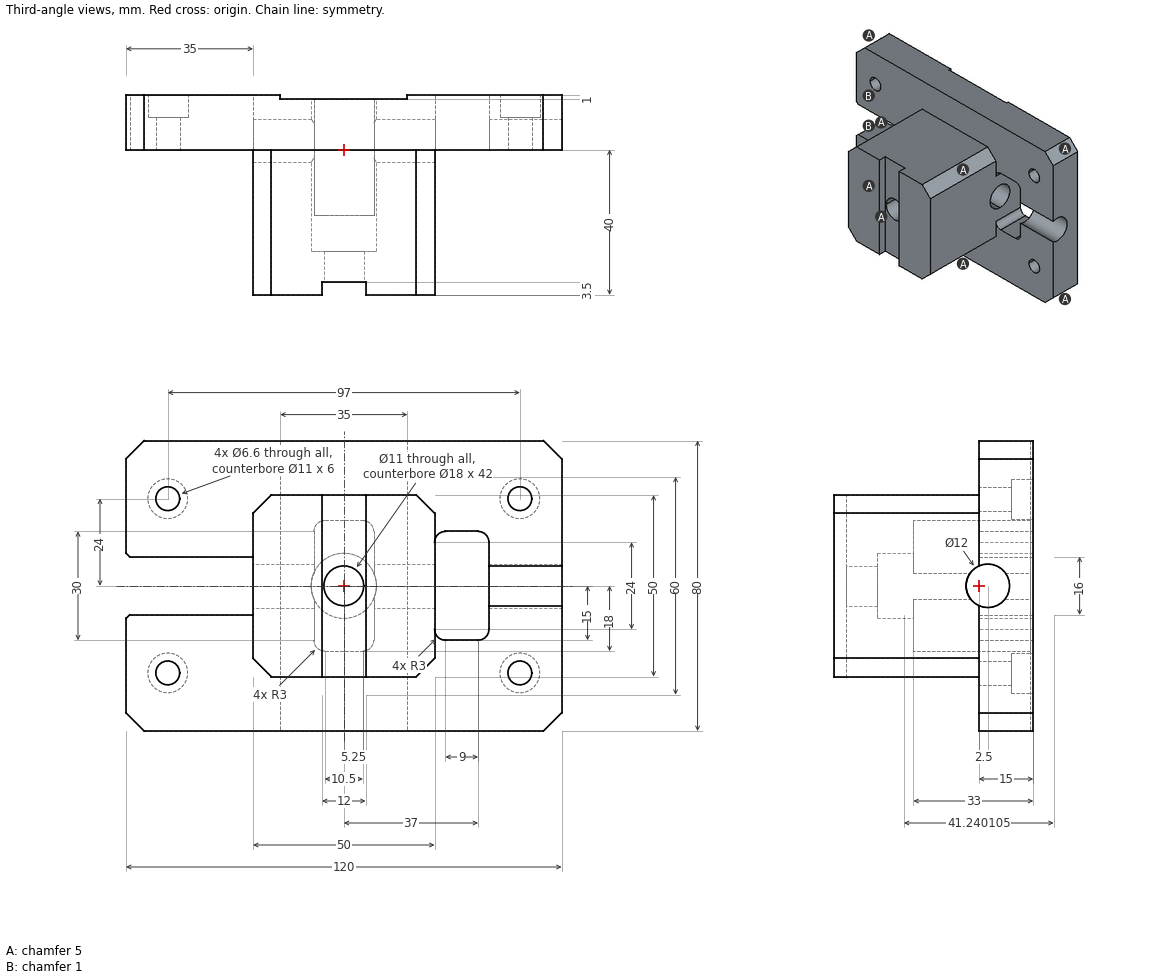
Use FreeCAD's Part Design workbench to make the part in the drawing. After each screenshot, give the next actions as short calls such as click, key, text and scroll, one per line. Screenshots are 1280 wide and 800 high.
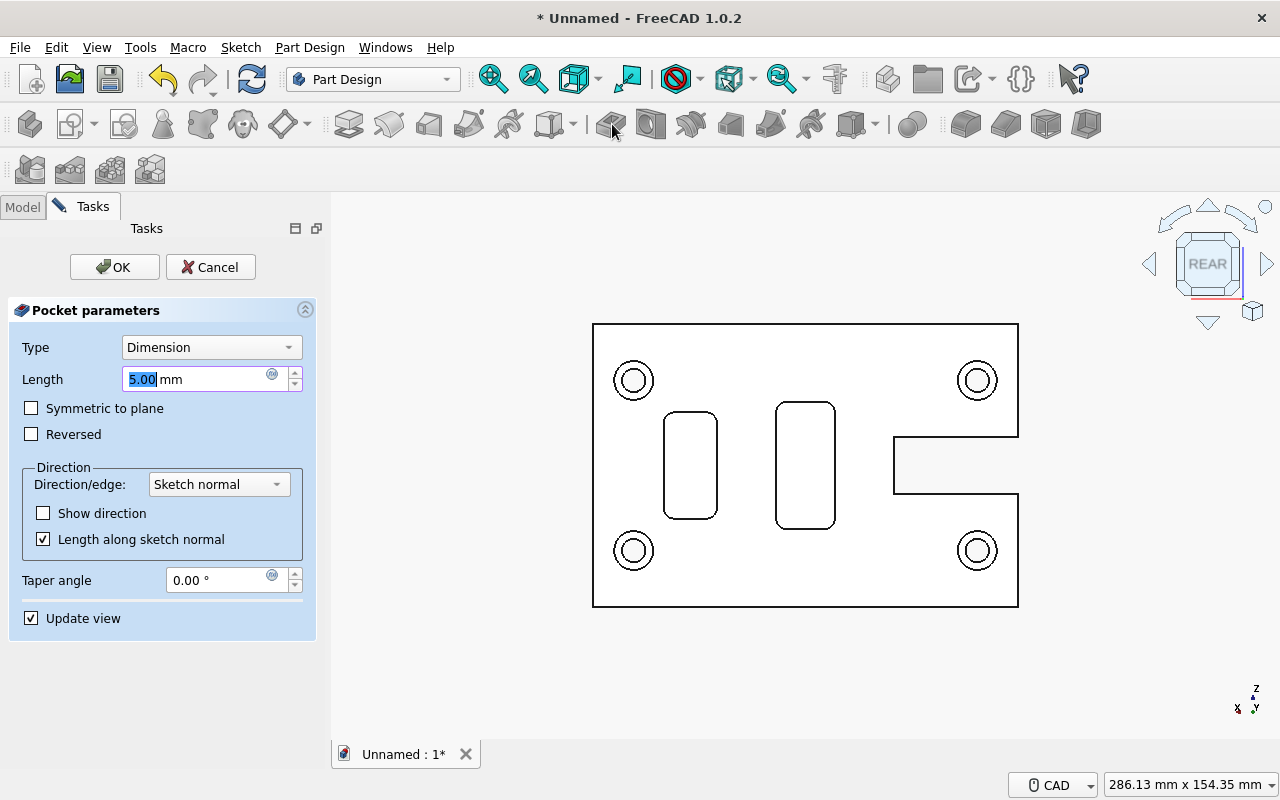
click(212, 348)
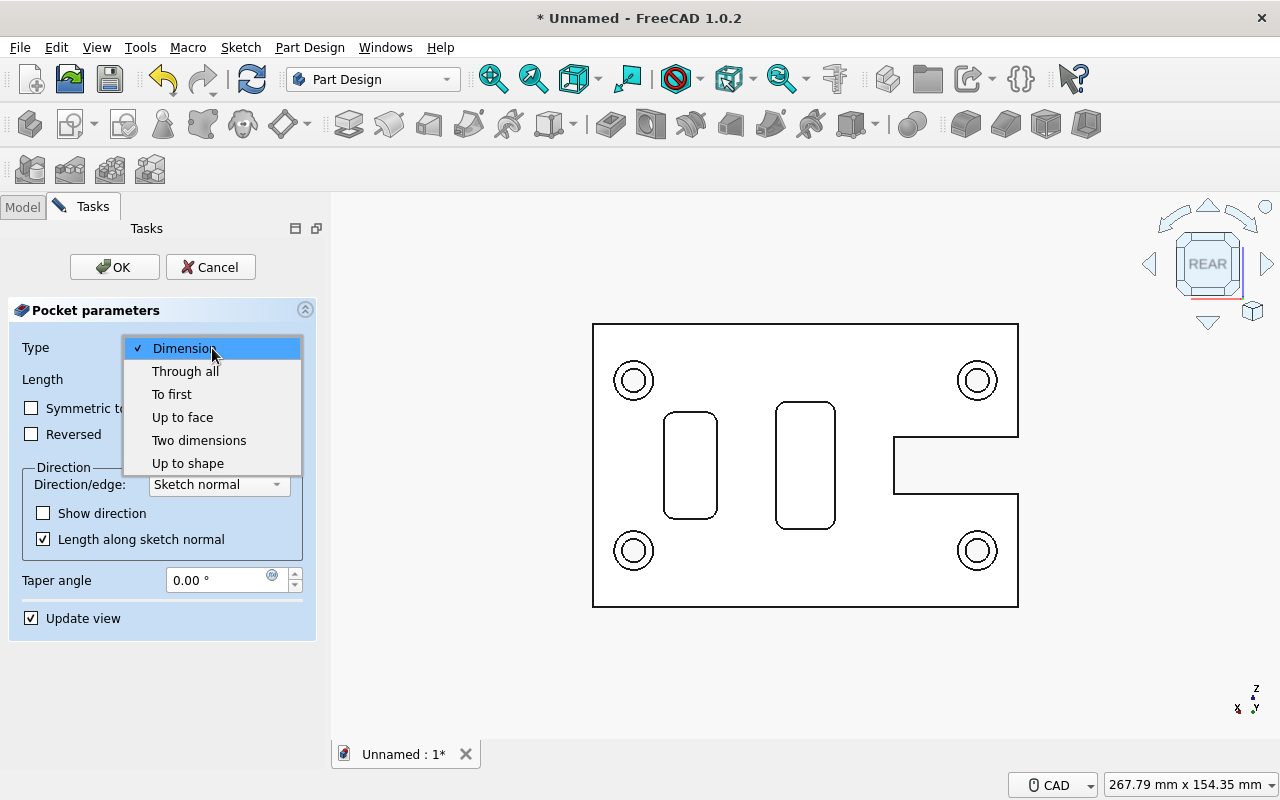
click(212, 372)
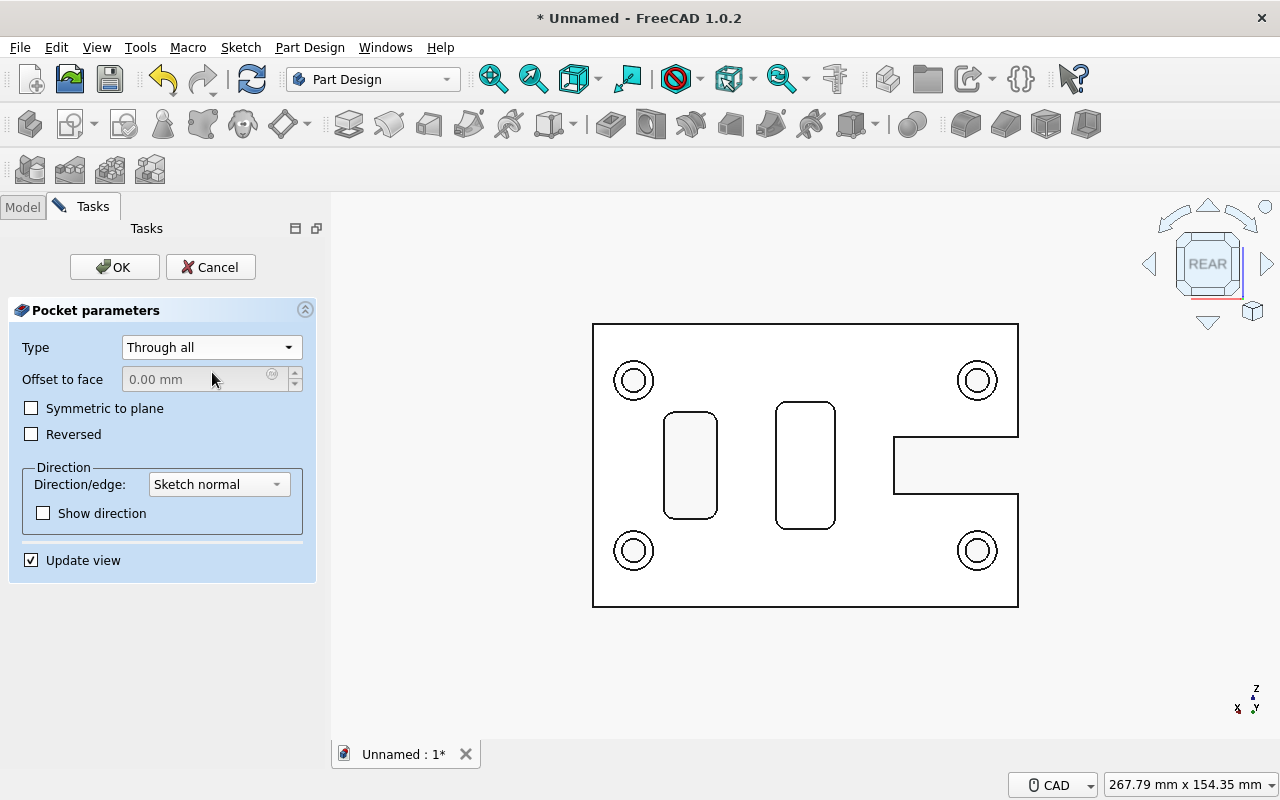
click(115, 267)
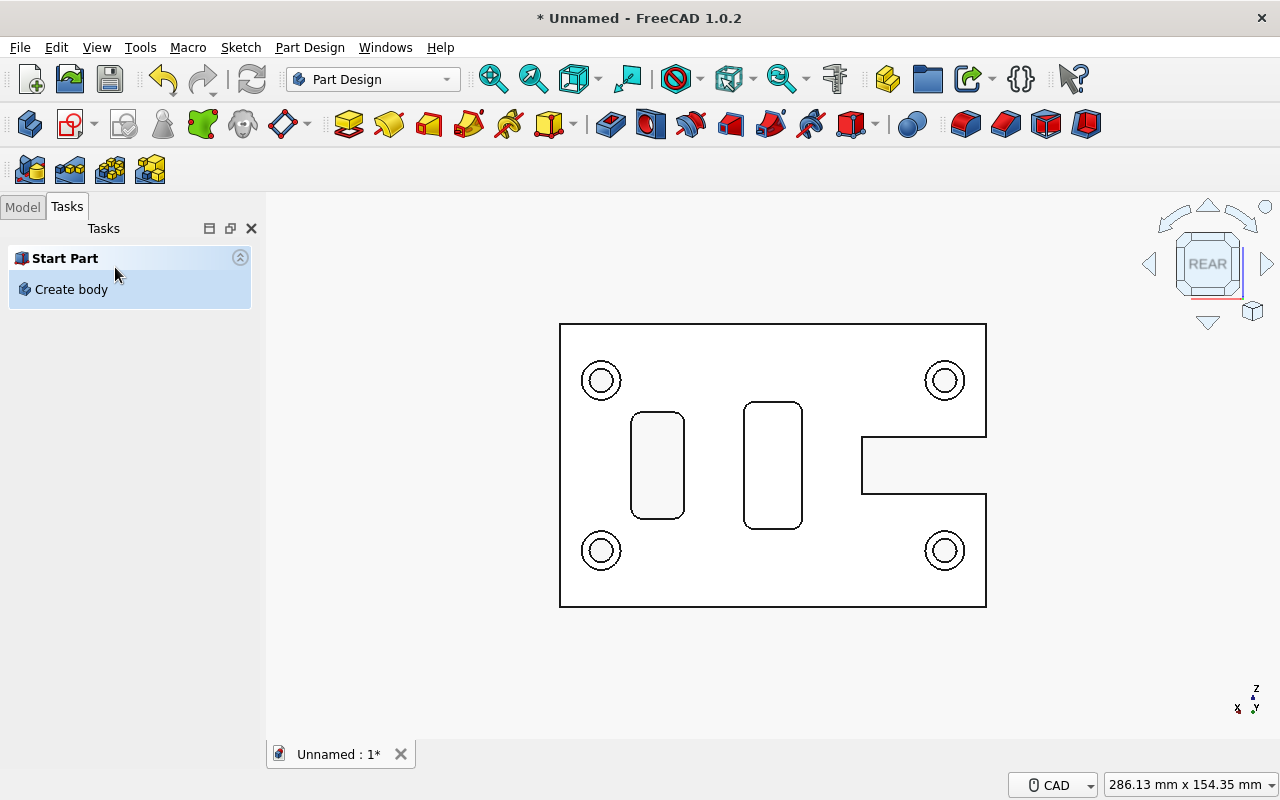
key(0)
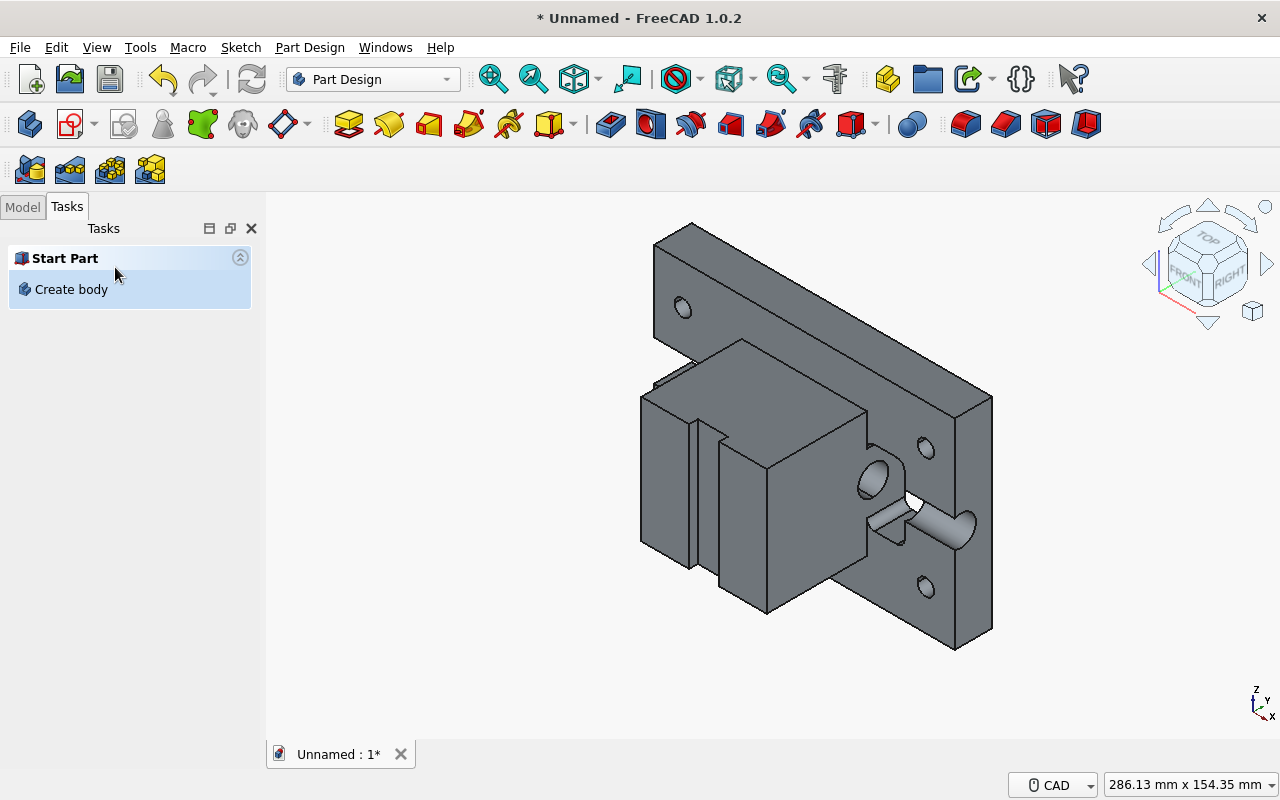
click(817, 439)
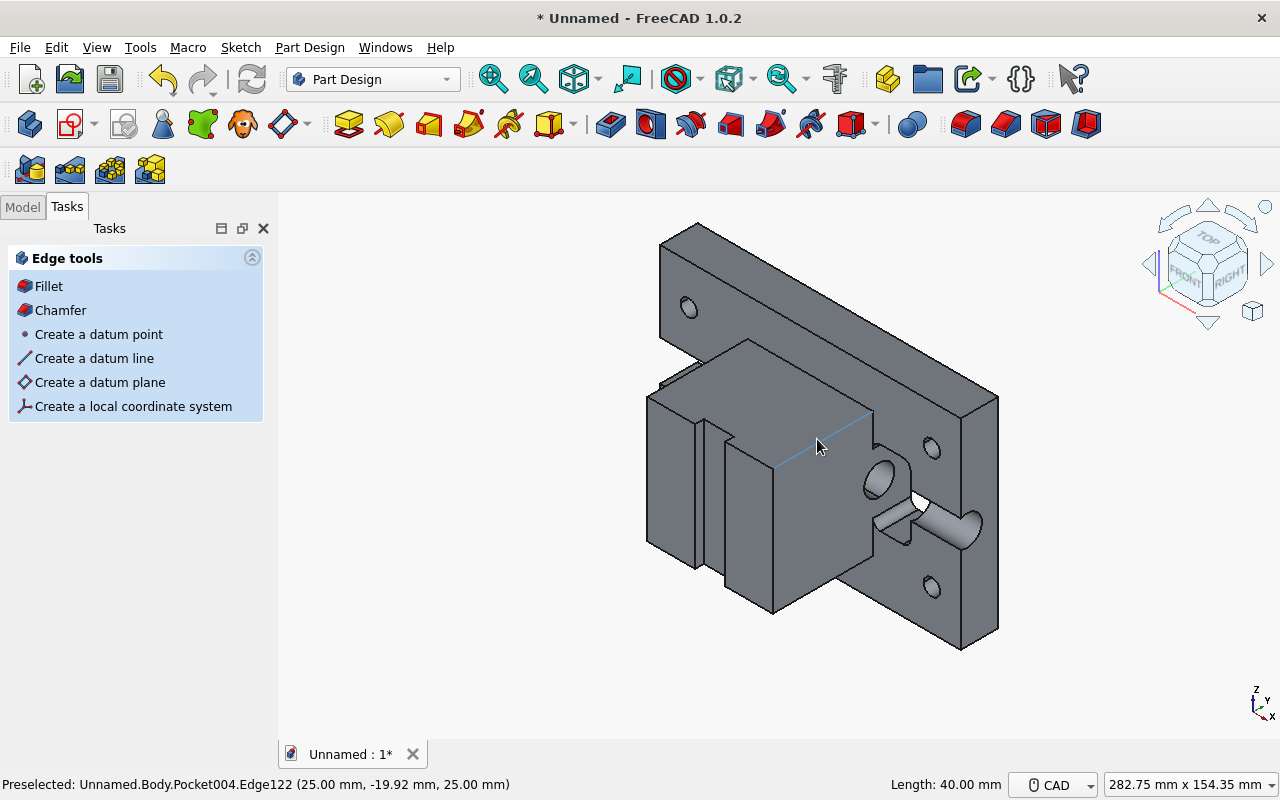
click(979, 407, ctrl)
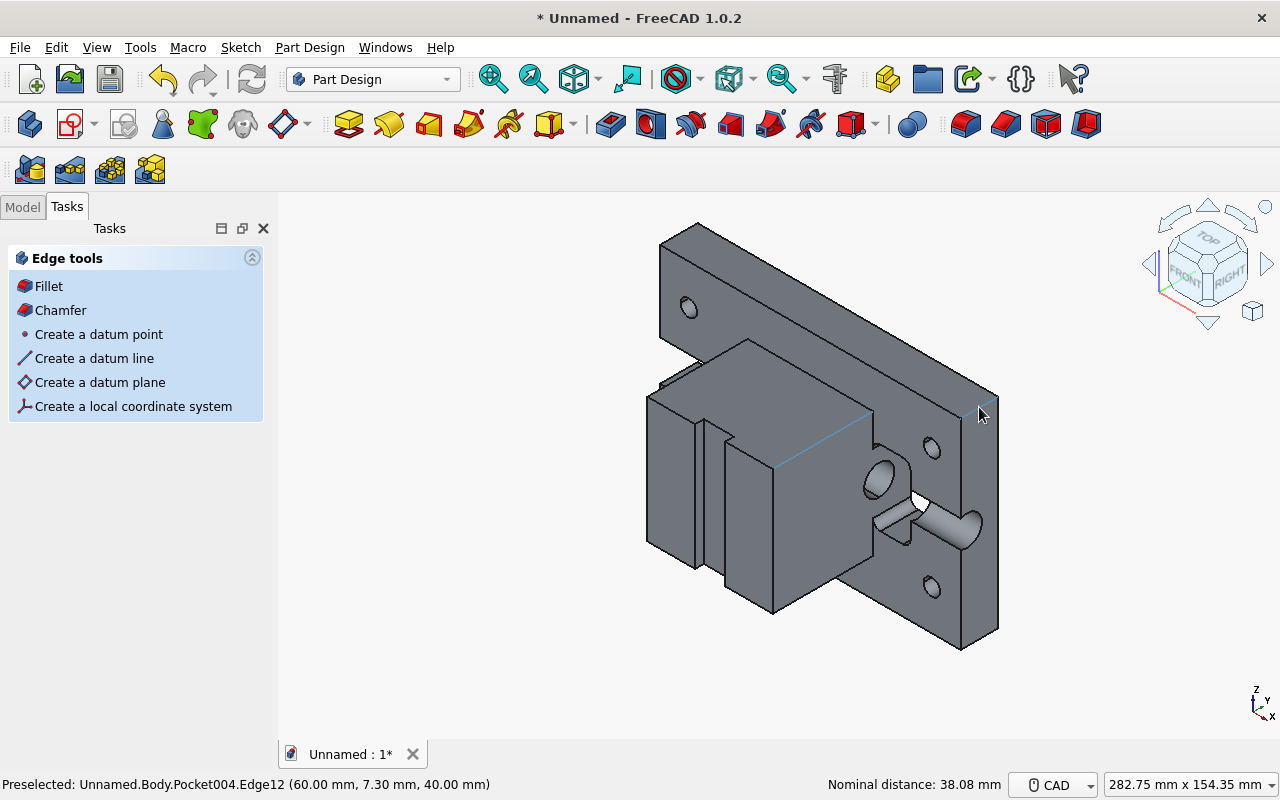
key(2)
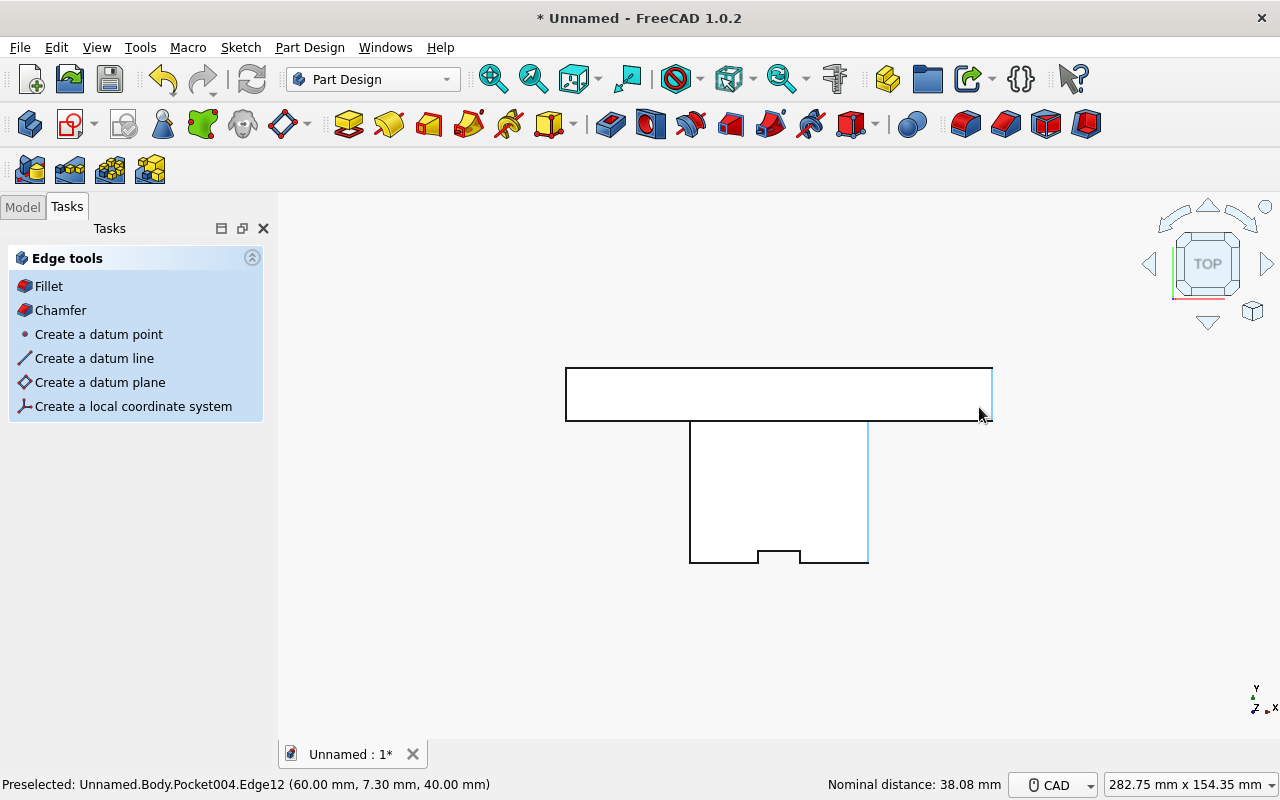
click(494, 80)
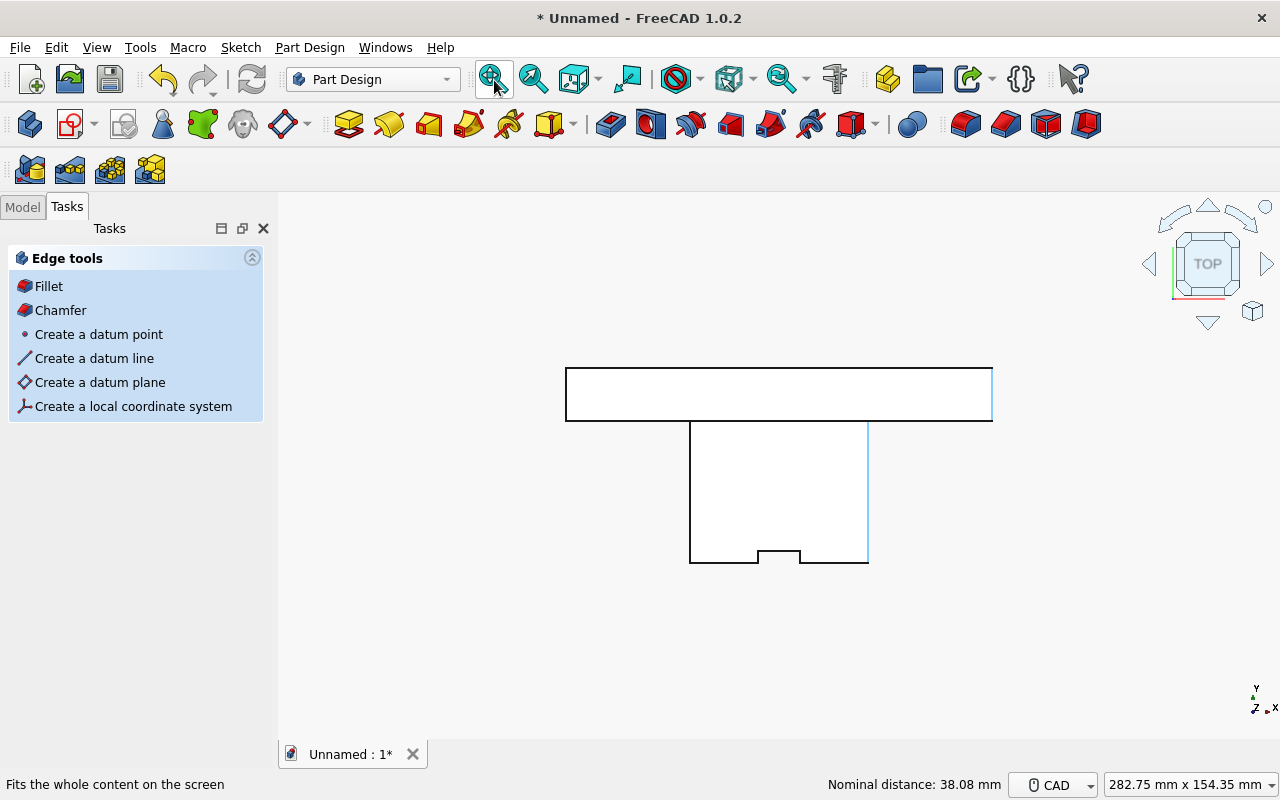
click(690, 491, ctrl)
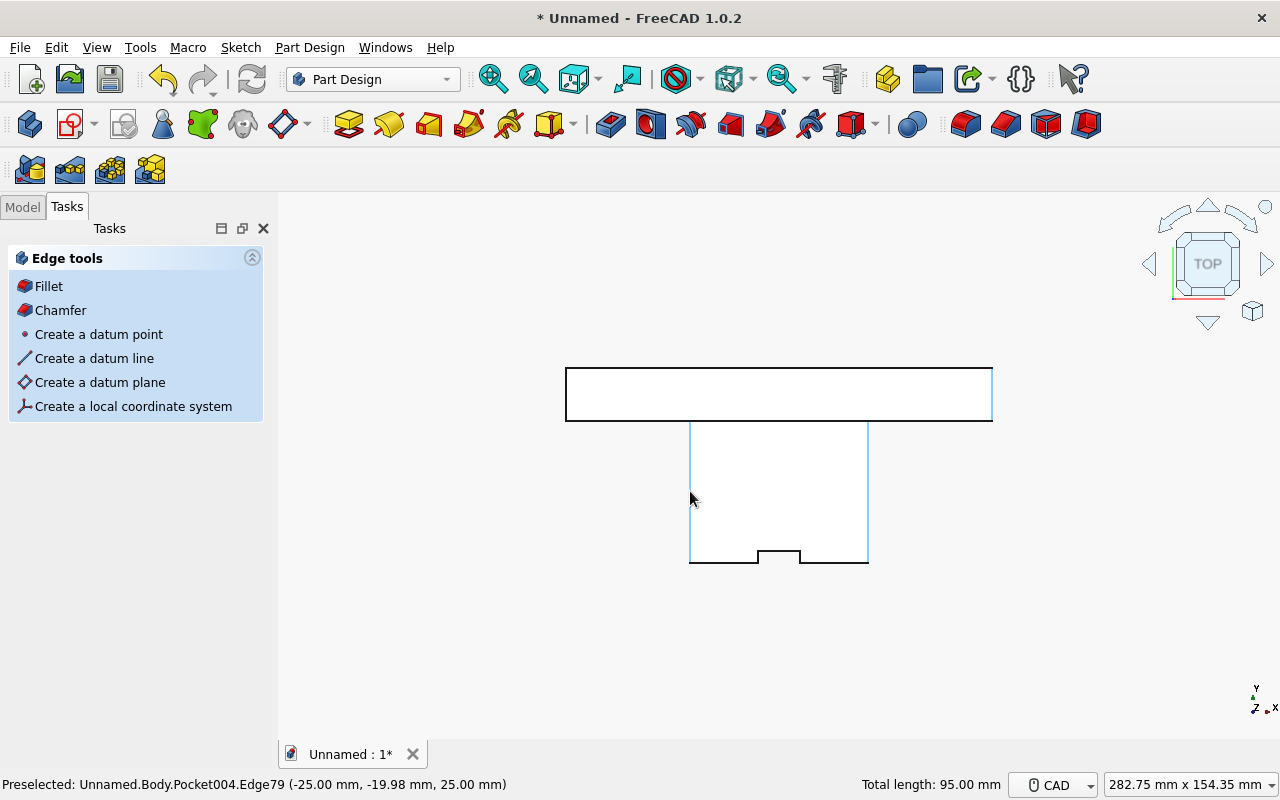
click(566, 394, ctrl)